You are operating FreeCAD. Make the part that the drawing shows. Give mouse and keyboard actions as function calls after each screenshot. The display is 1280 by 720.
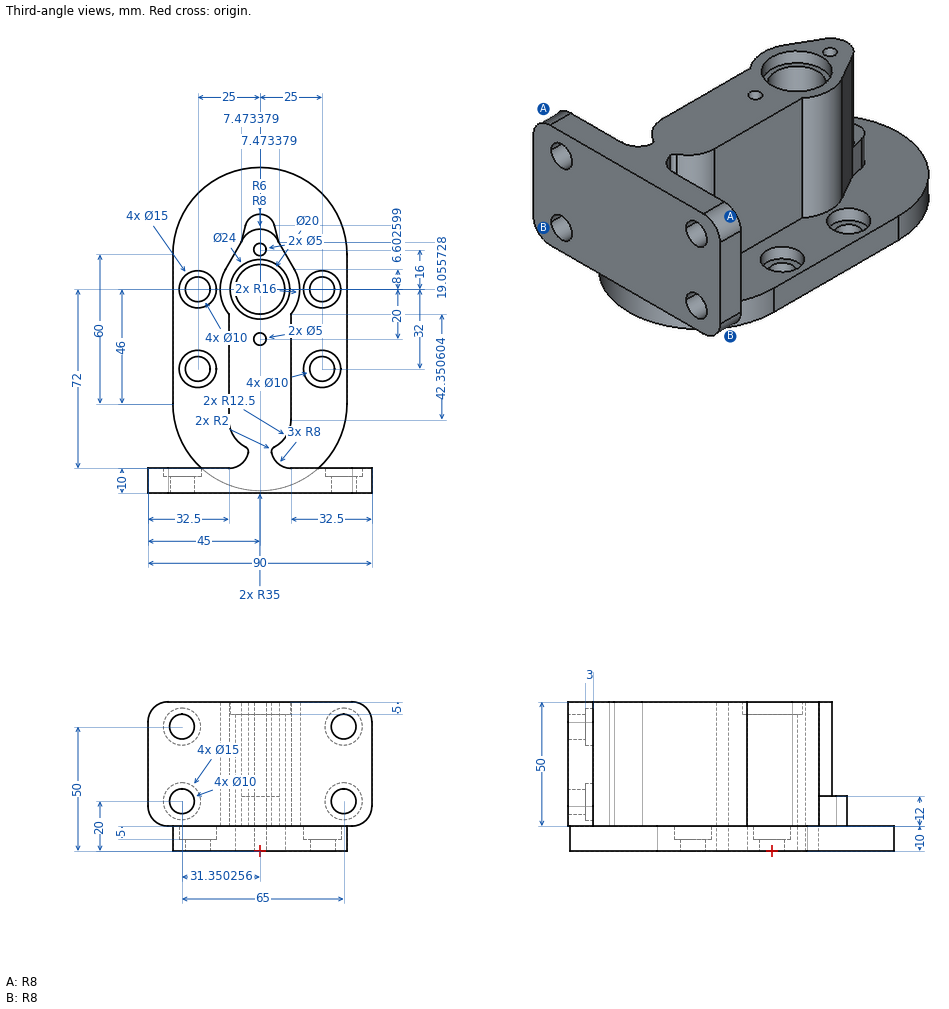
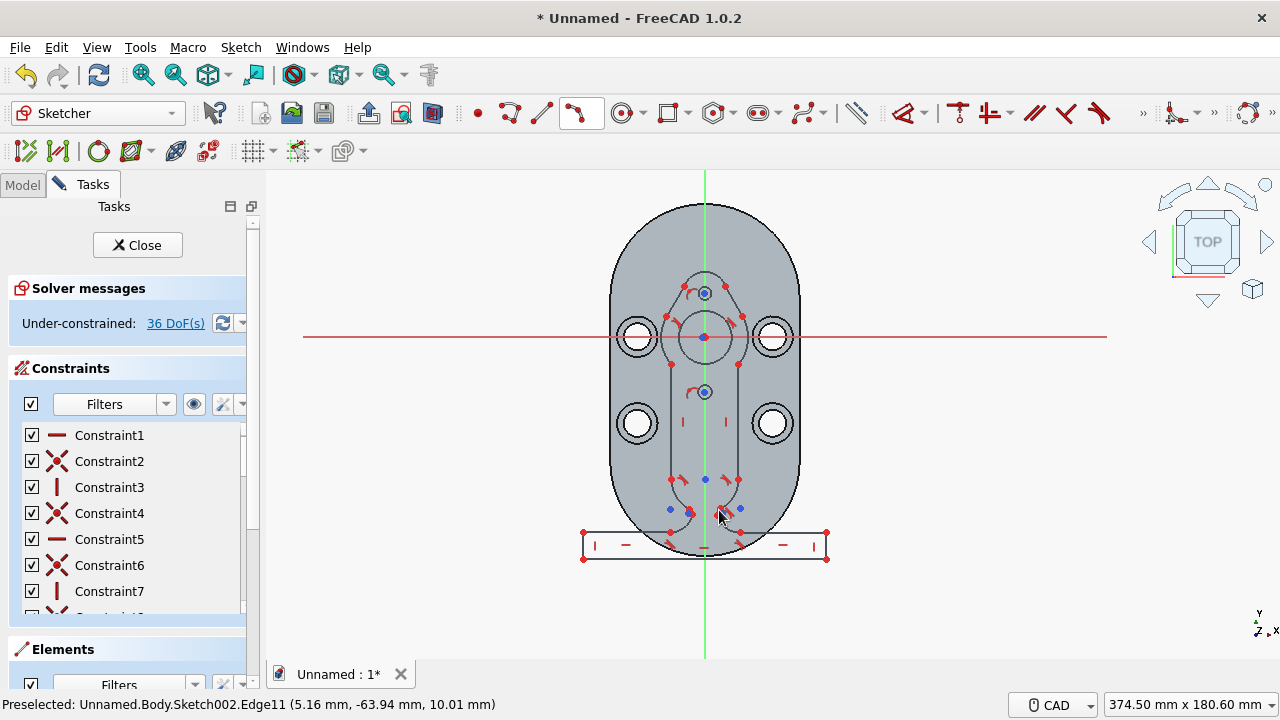
scroll(729, 502, up, 2)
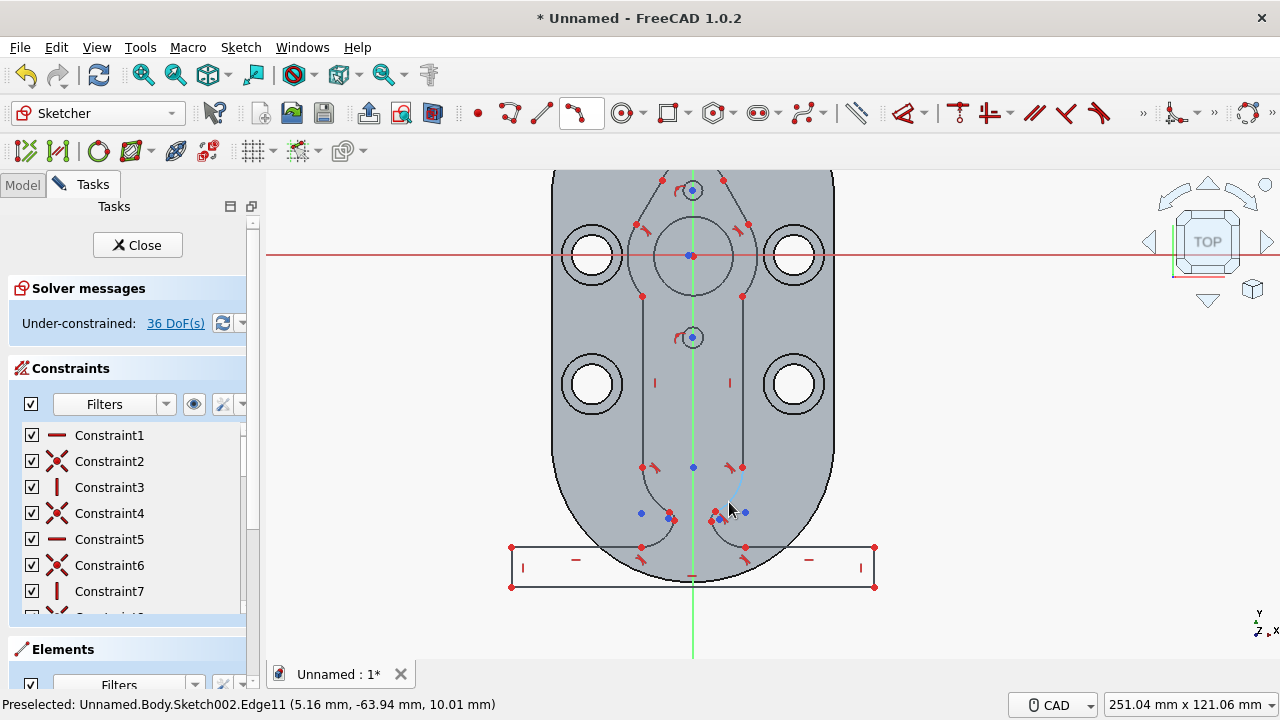
click(729, 502)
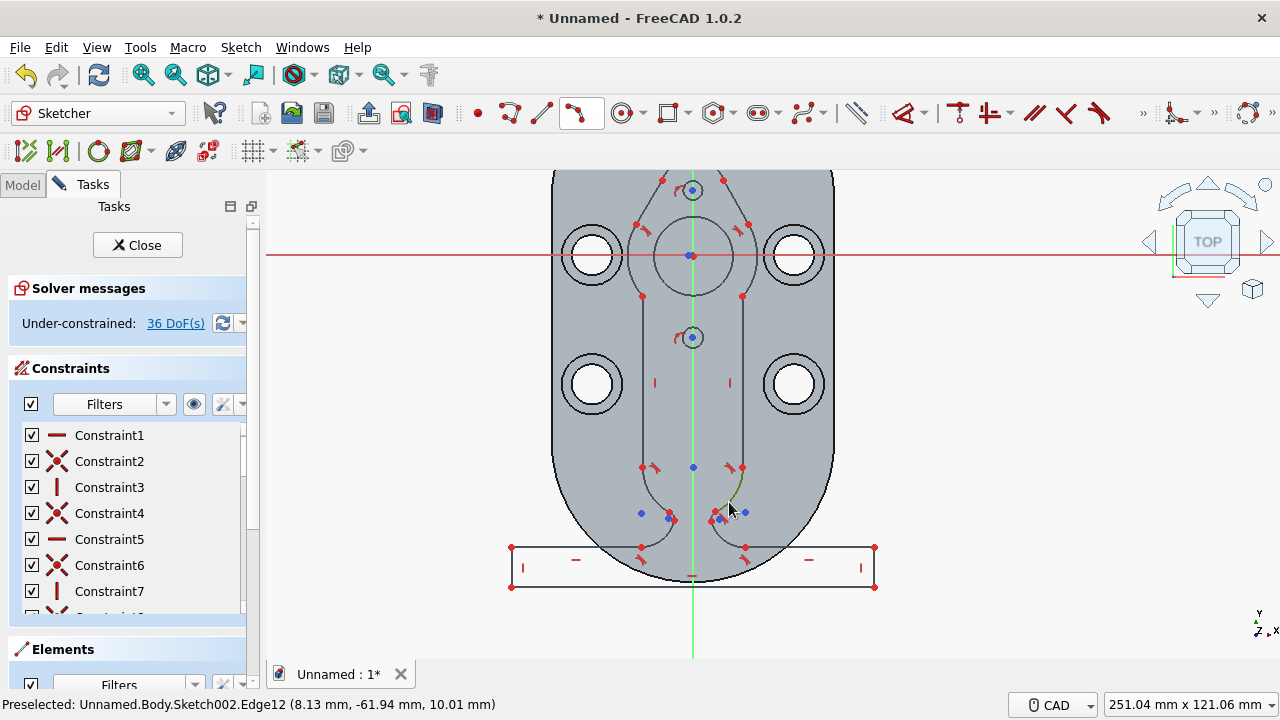
click(1100, 114)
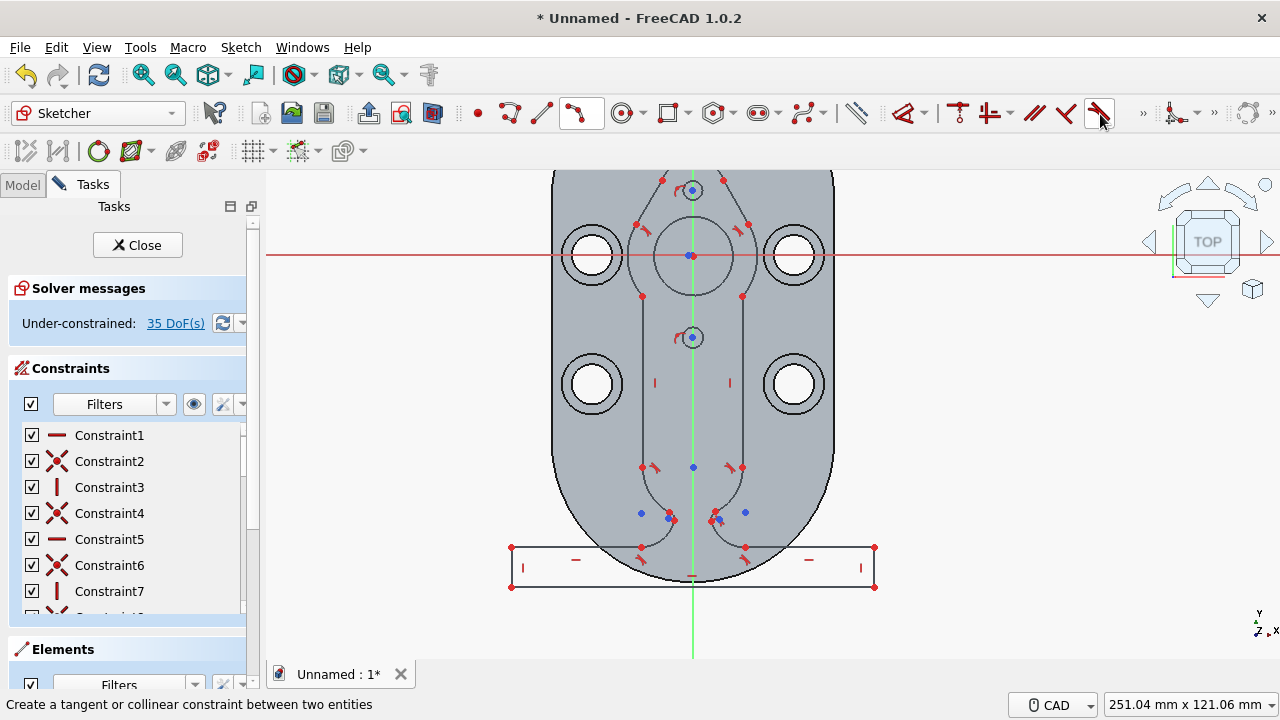
click(646, 484)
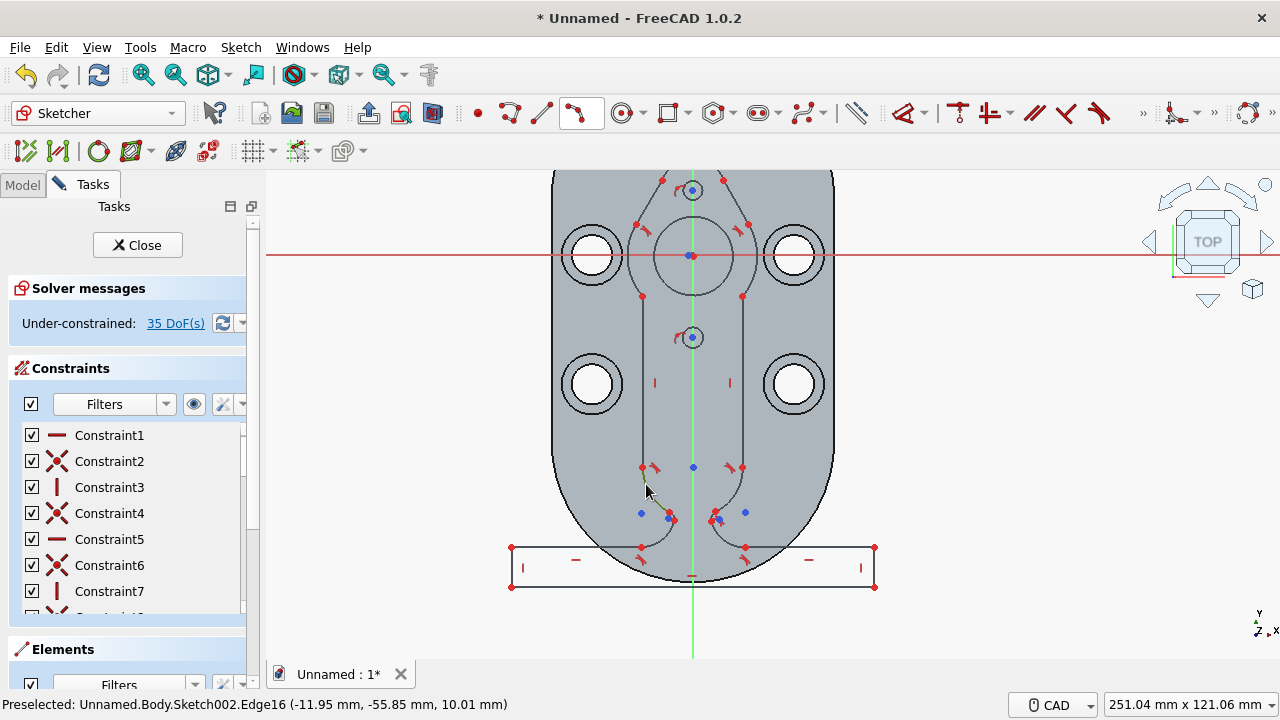
scroll(674, 516, up, 5)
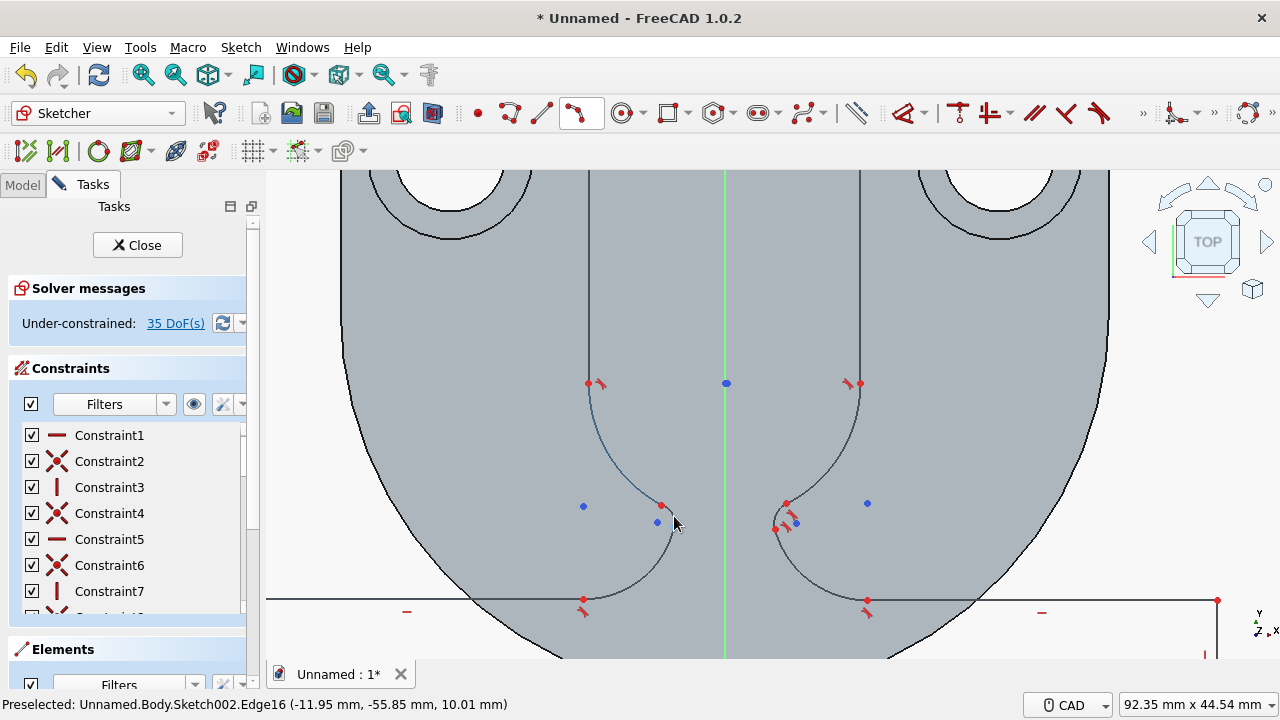
click(673, 514)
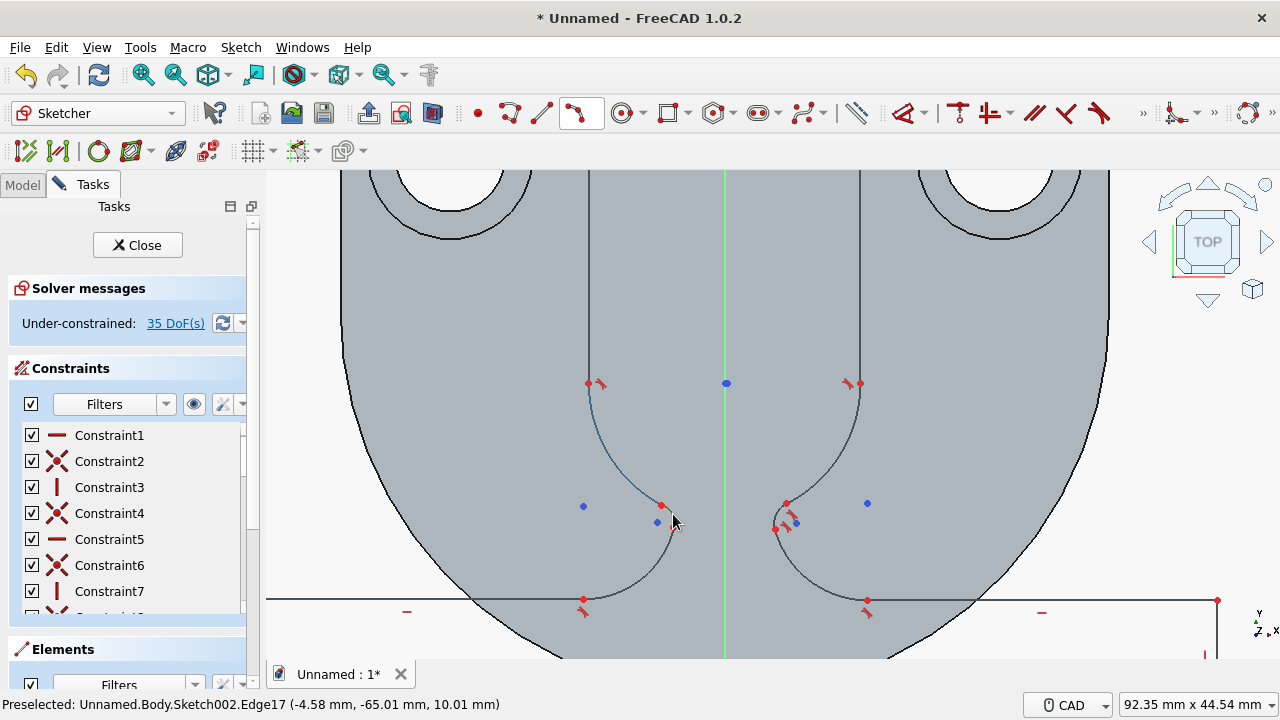
click(1100, 114)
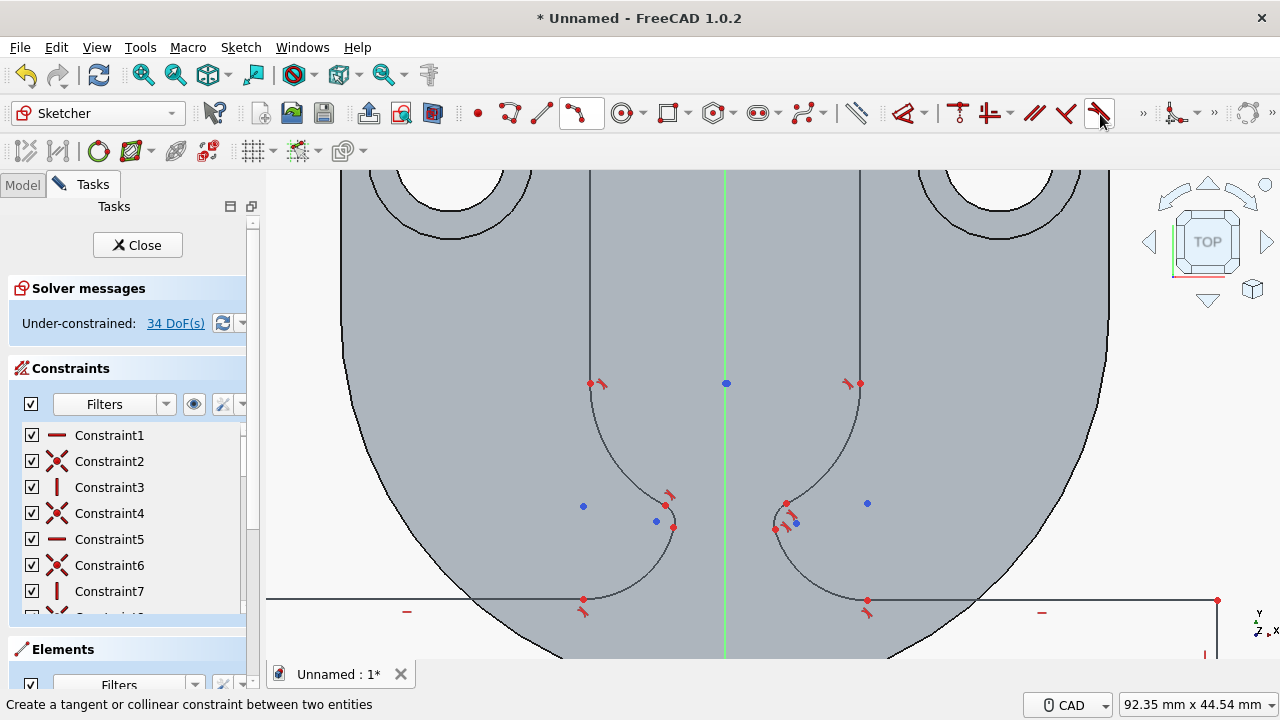
click(674, 515)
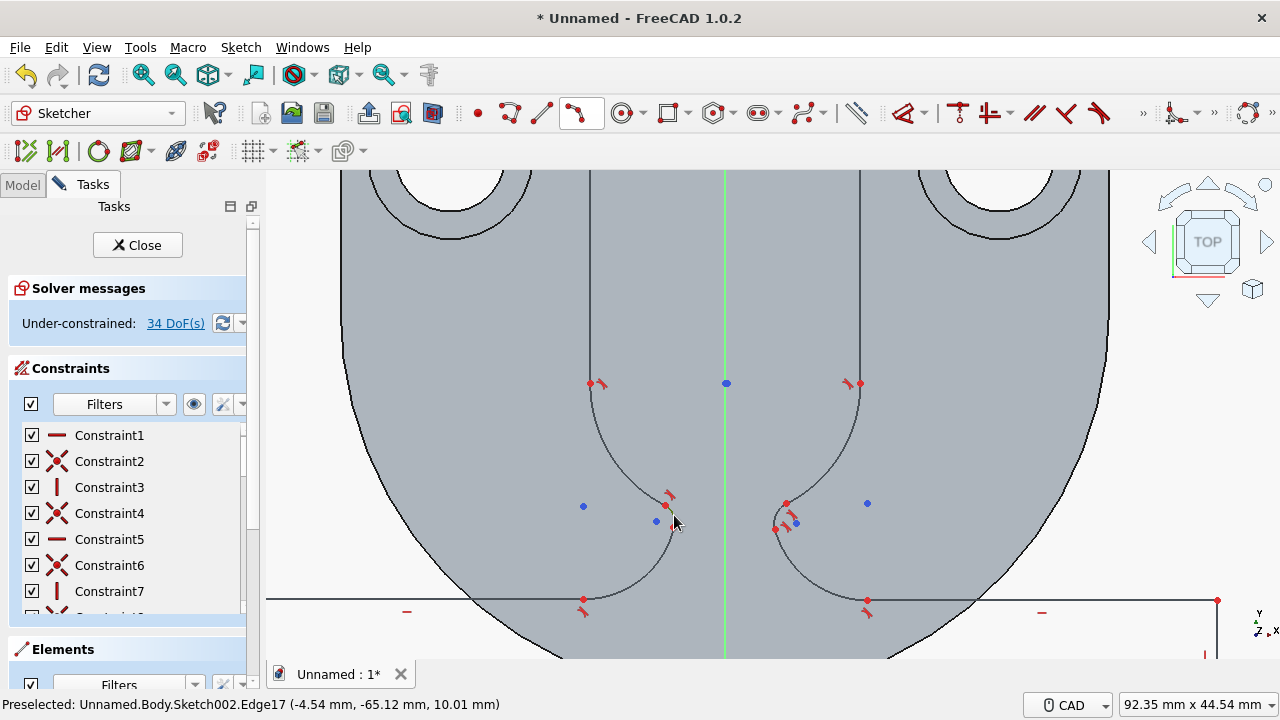
click(620, 592)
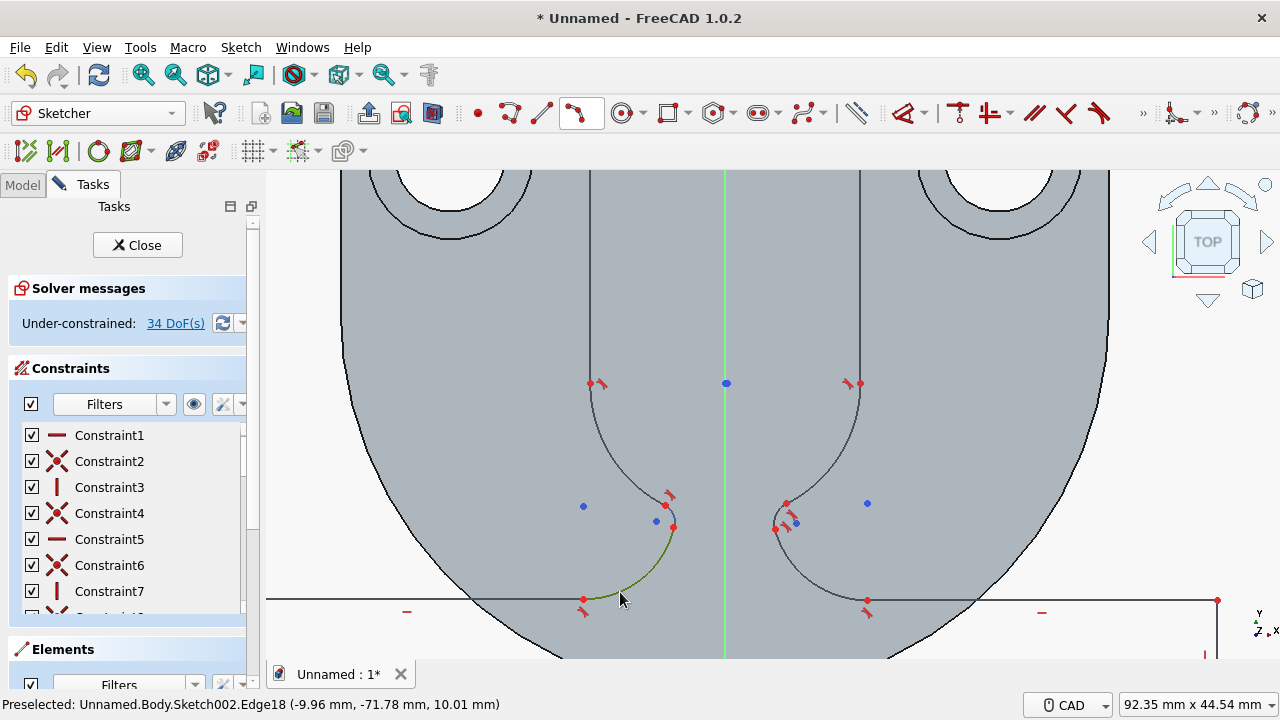
click(1100, 114)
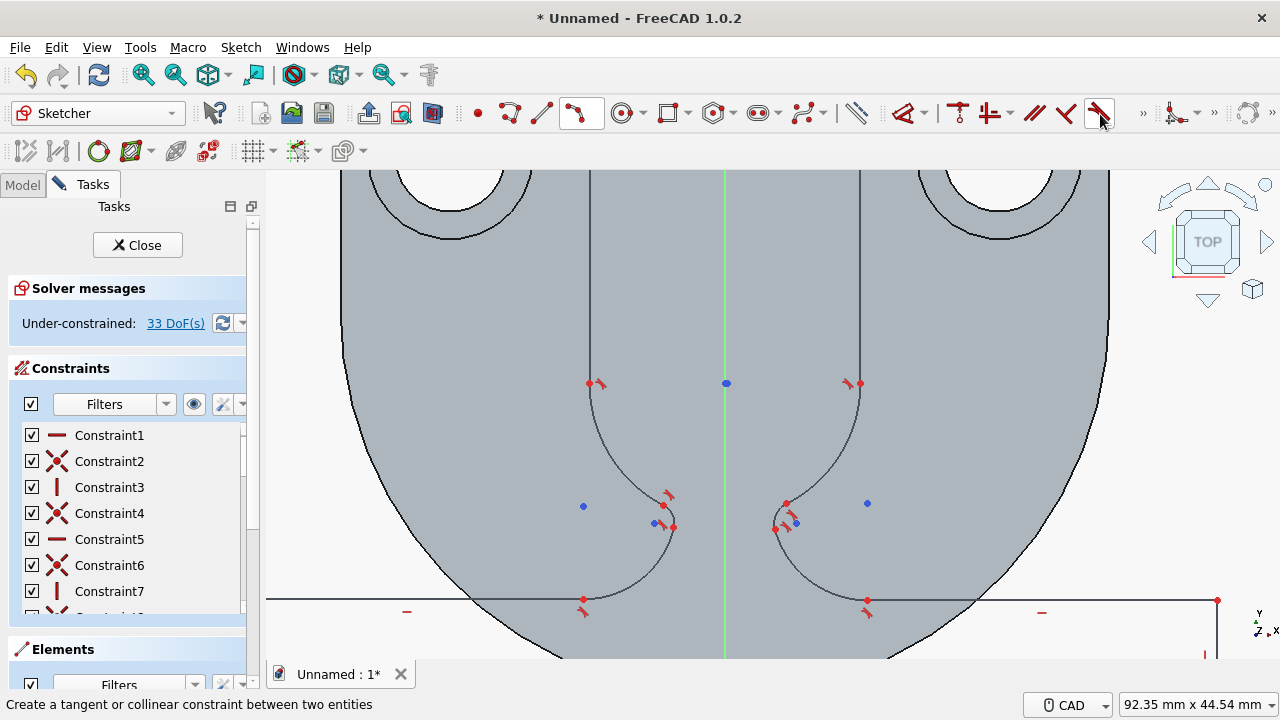
scroll(698, 510, down, 7)